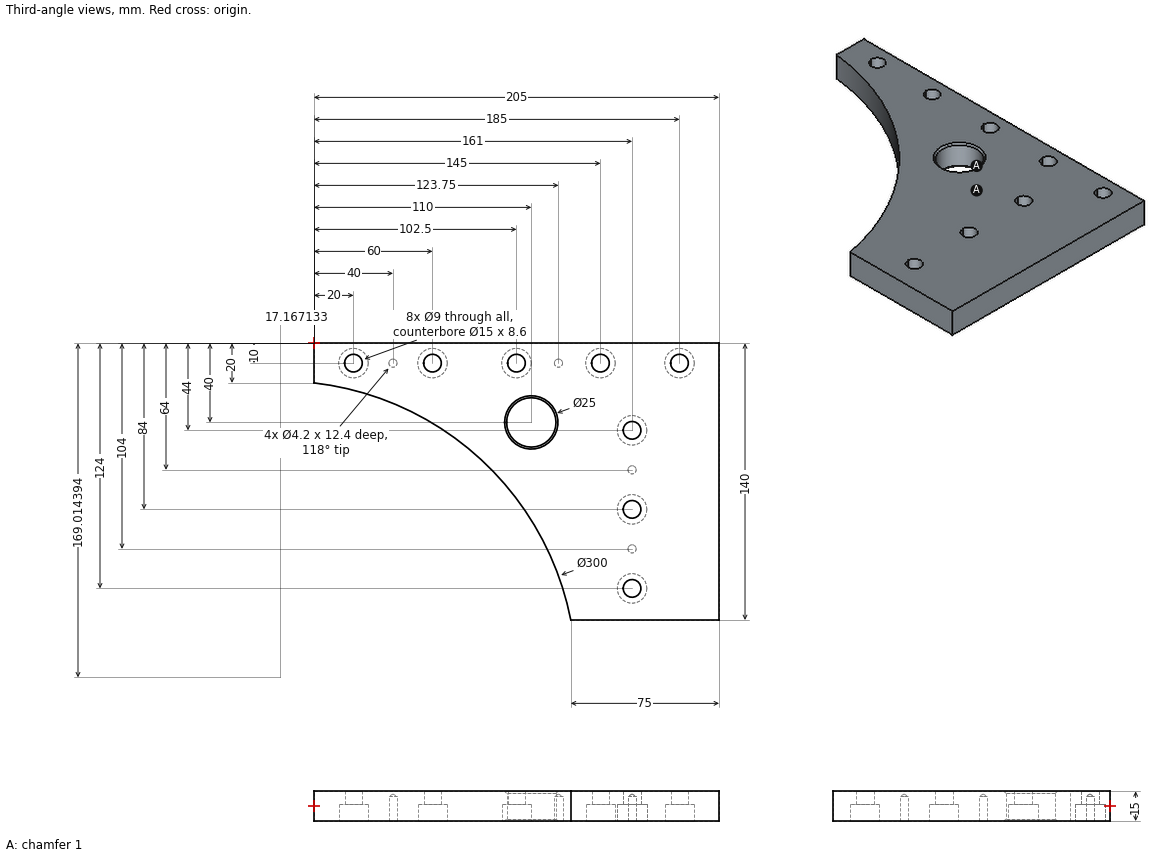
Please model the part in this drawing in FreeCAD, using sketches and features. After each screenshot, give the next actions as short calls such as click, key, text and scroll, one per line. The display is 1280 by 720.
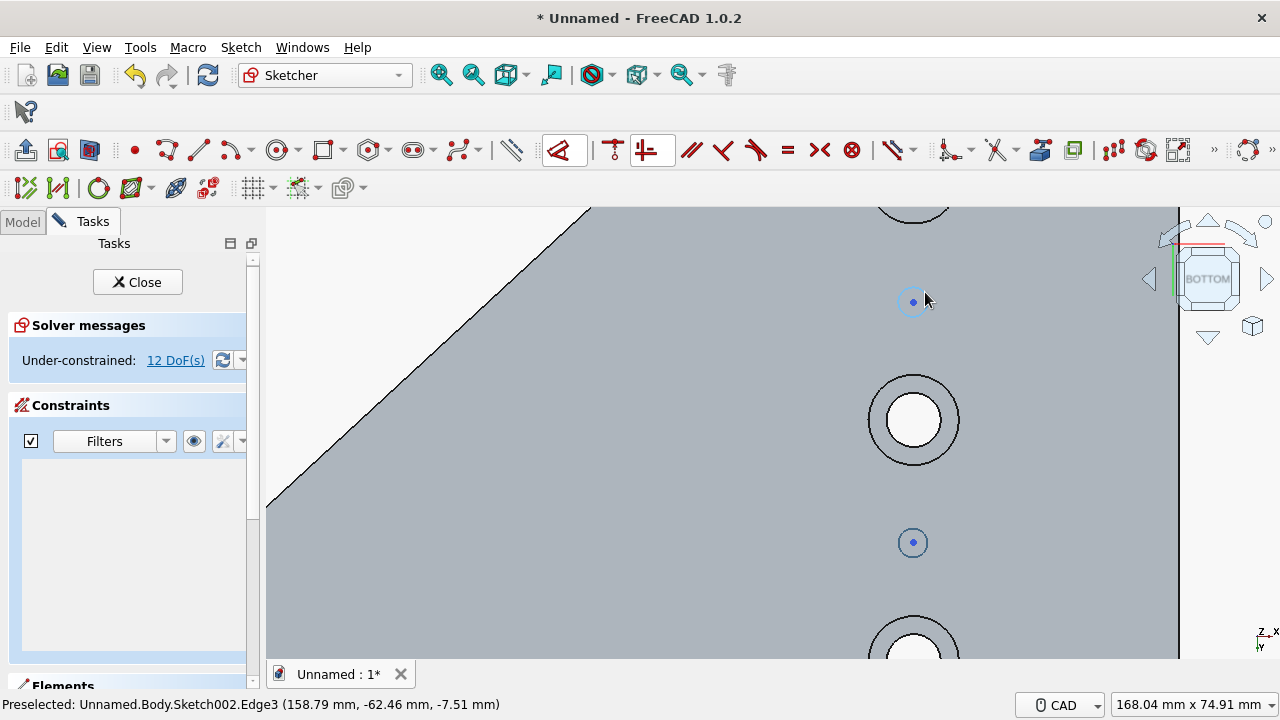
click(923, 292)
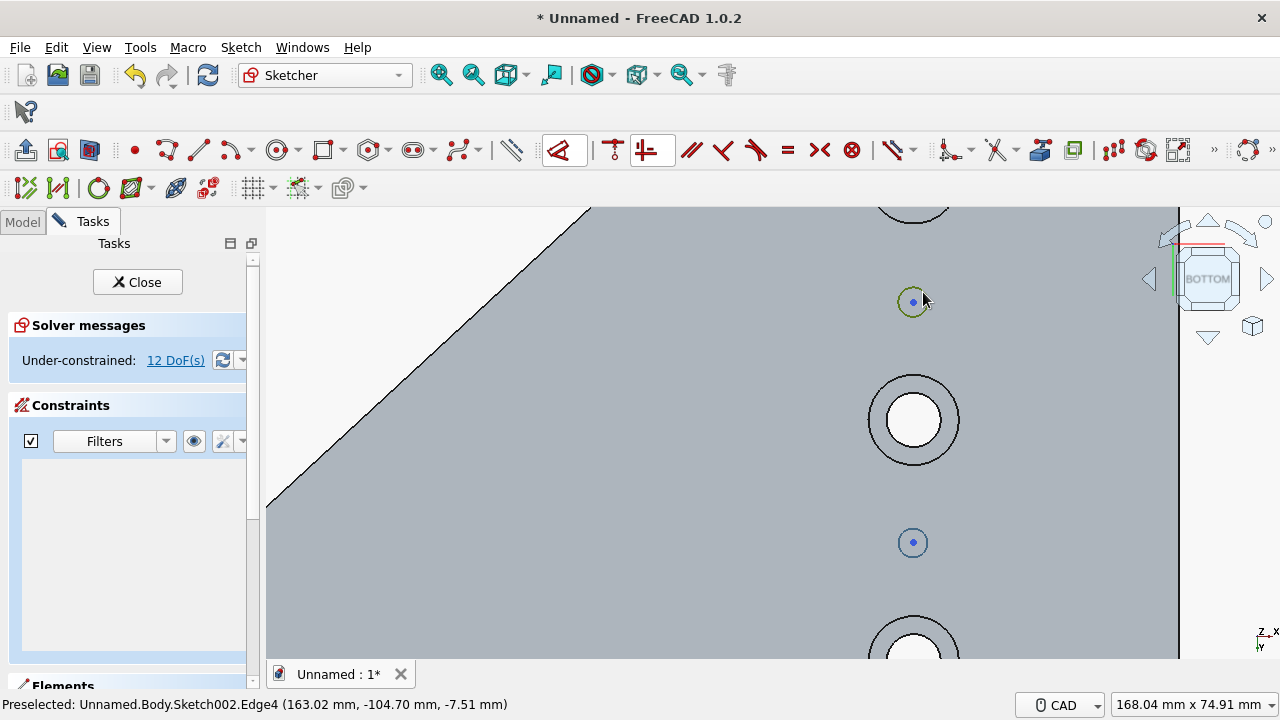
click(788, 150)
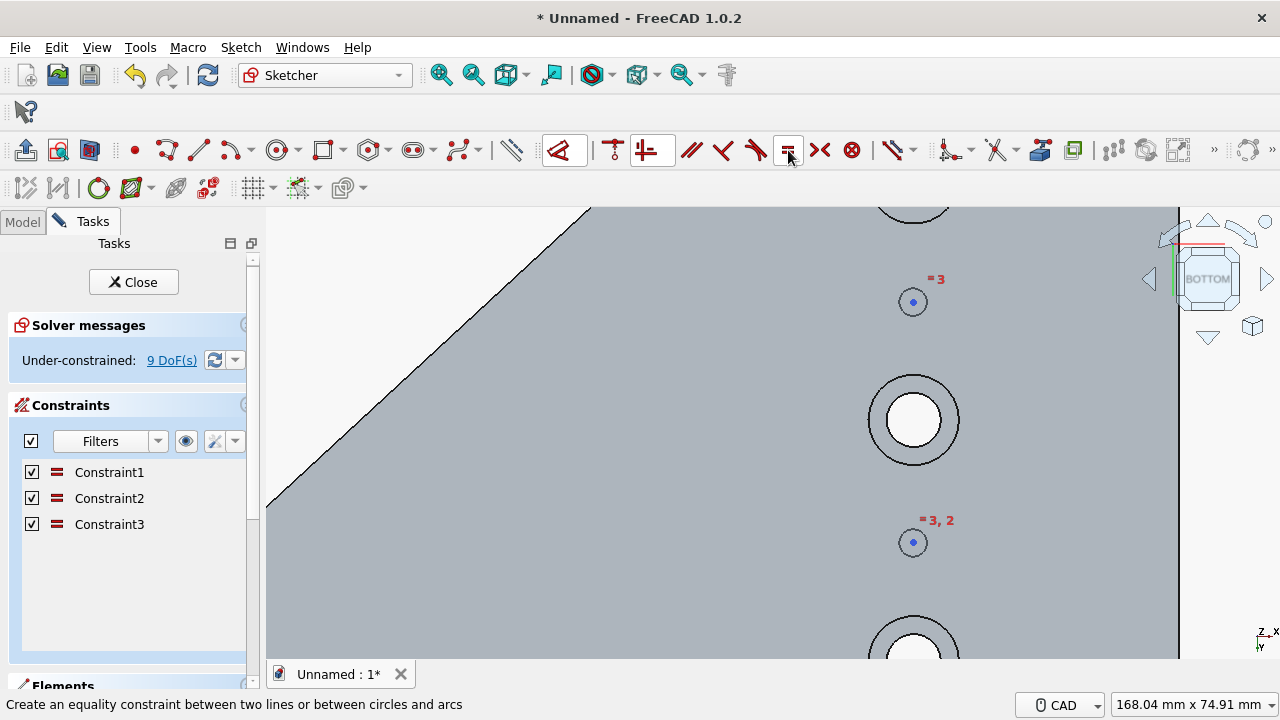
scroll(925, 291, down, 4)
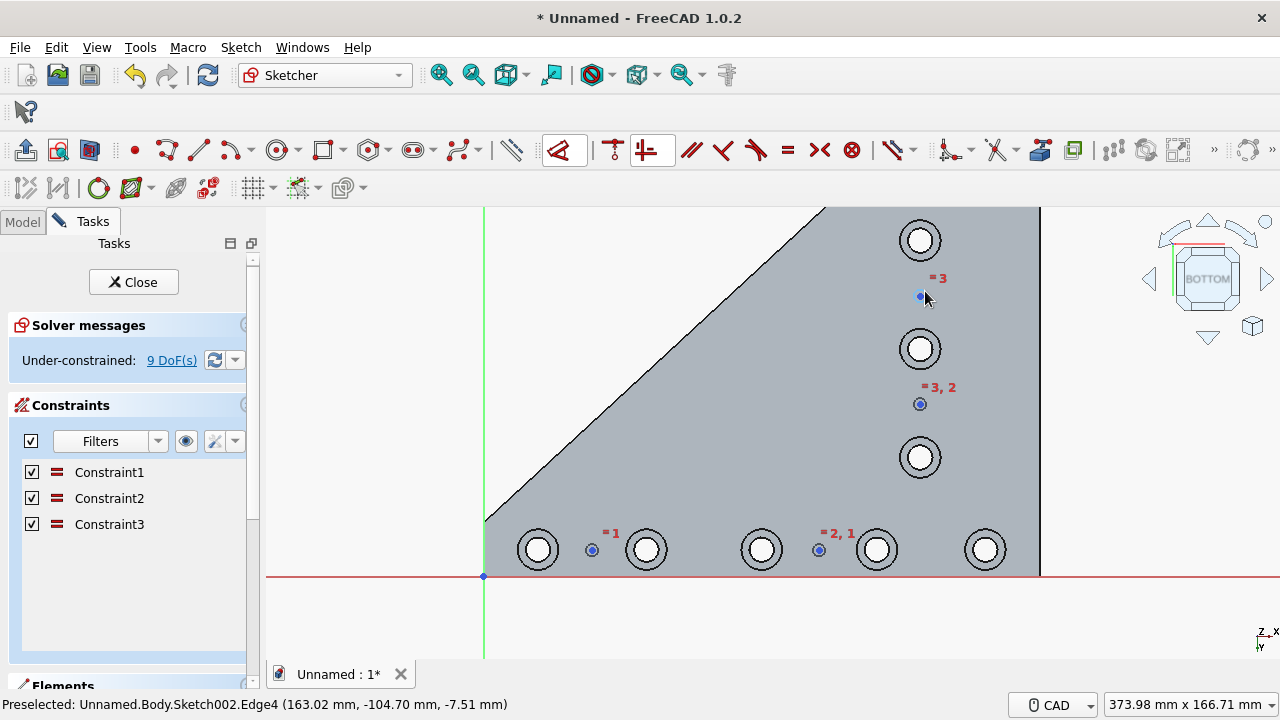
scroll(596, 546, up, 7)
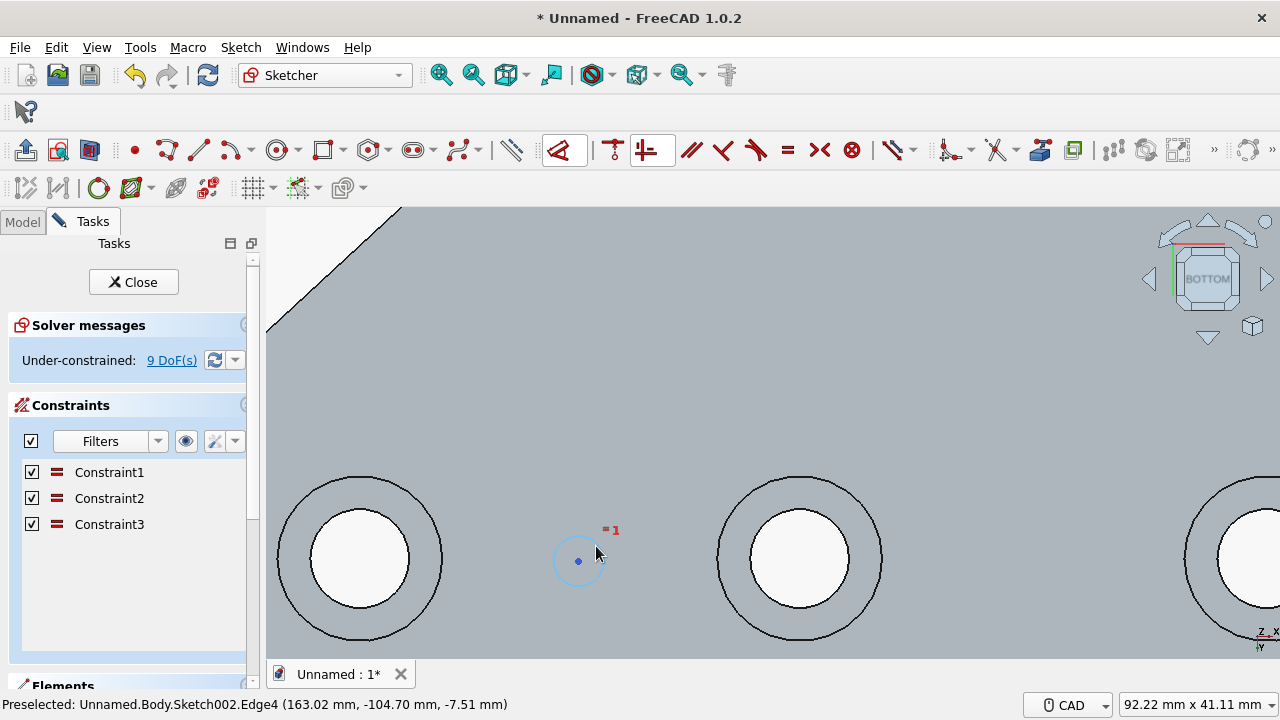
click(596, 544)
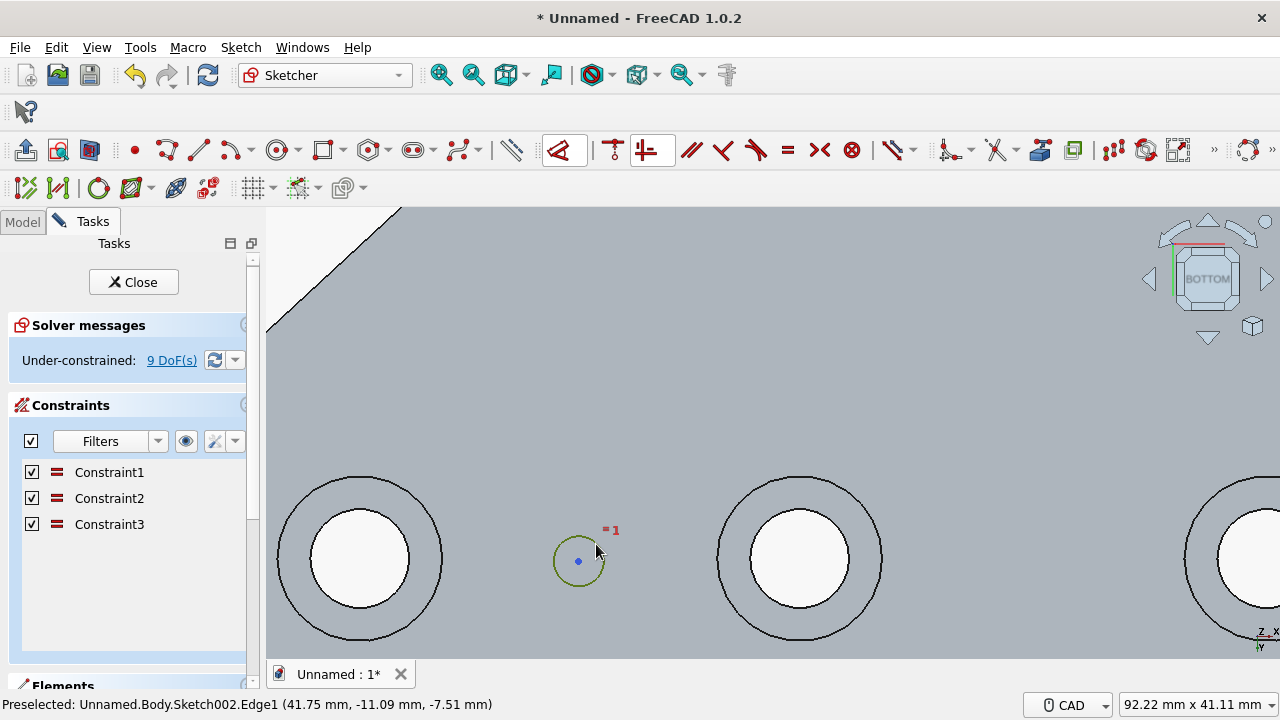
click(582, 150)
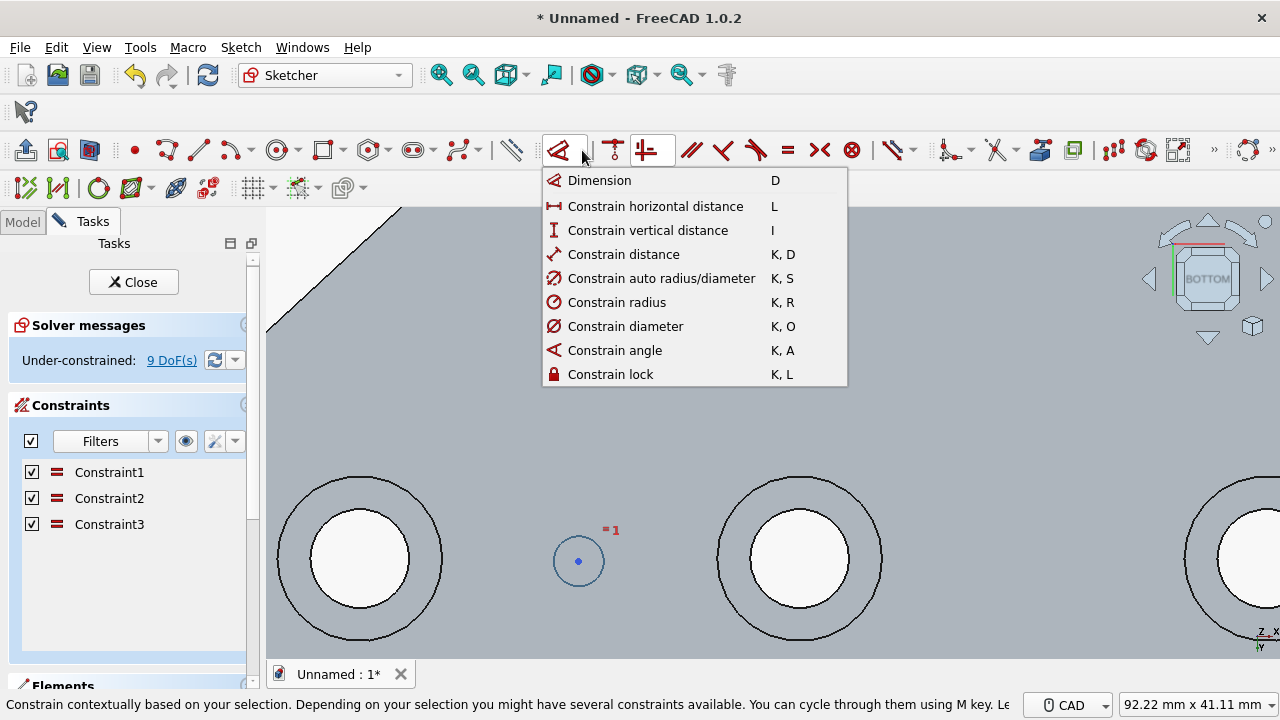
click(695, 326)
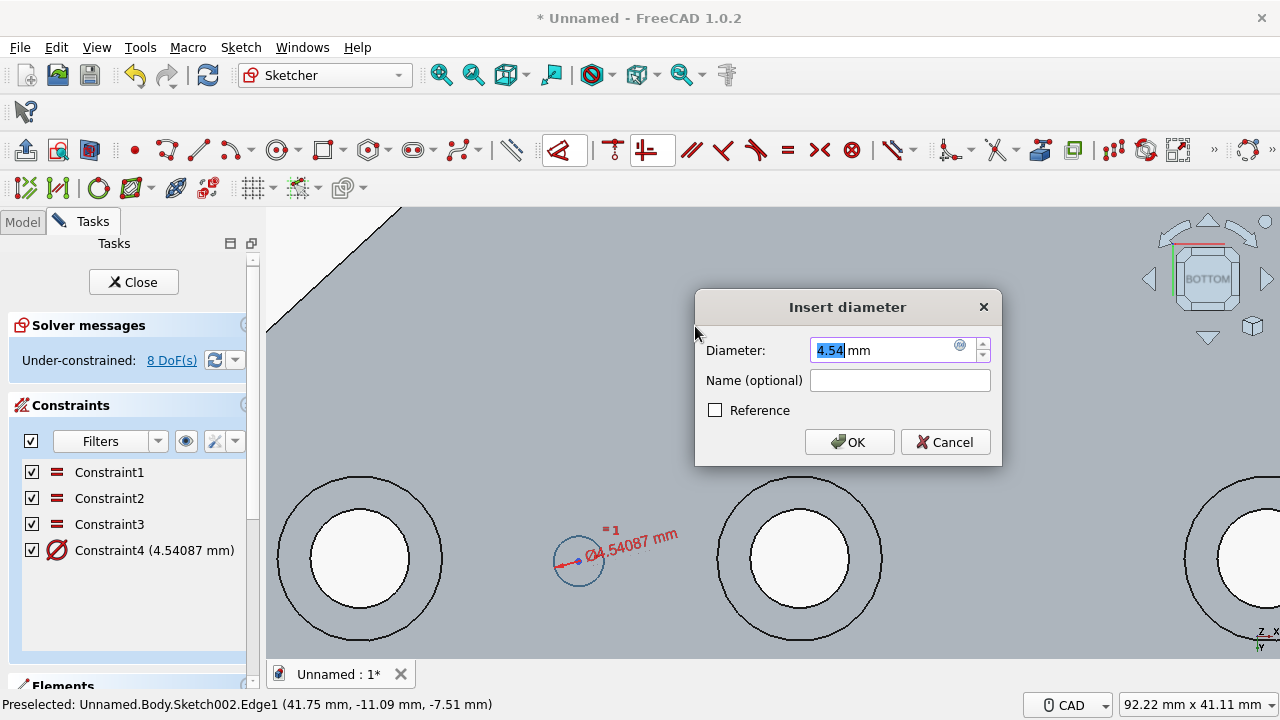
text(4.2)
key(Return)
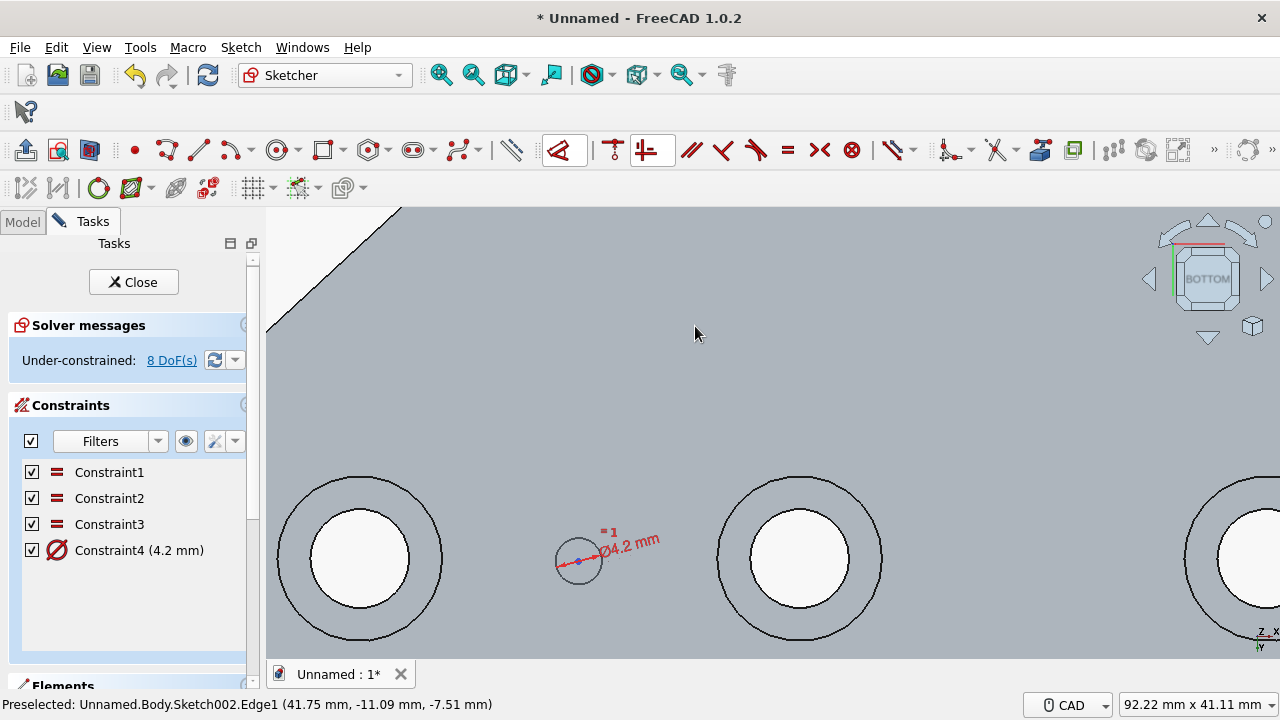
scroll(596, 547, down, 7)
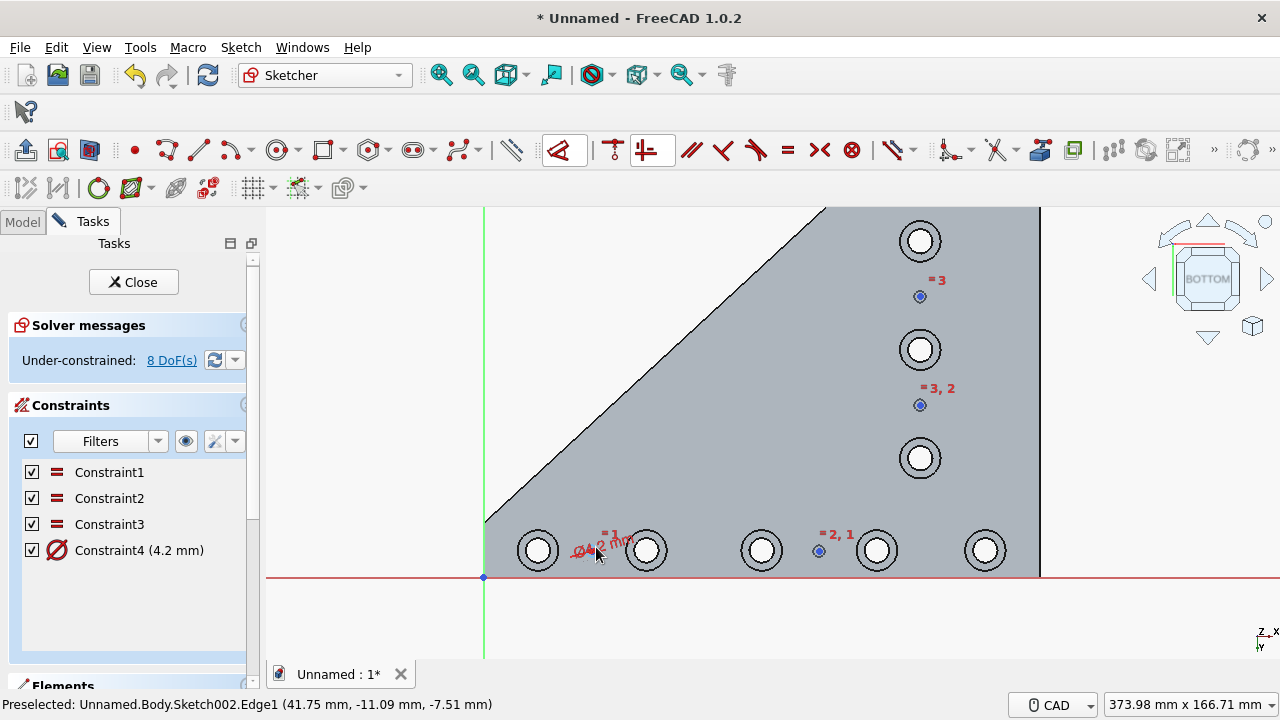
click(592, 551)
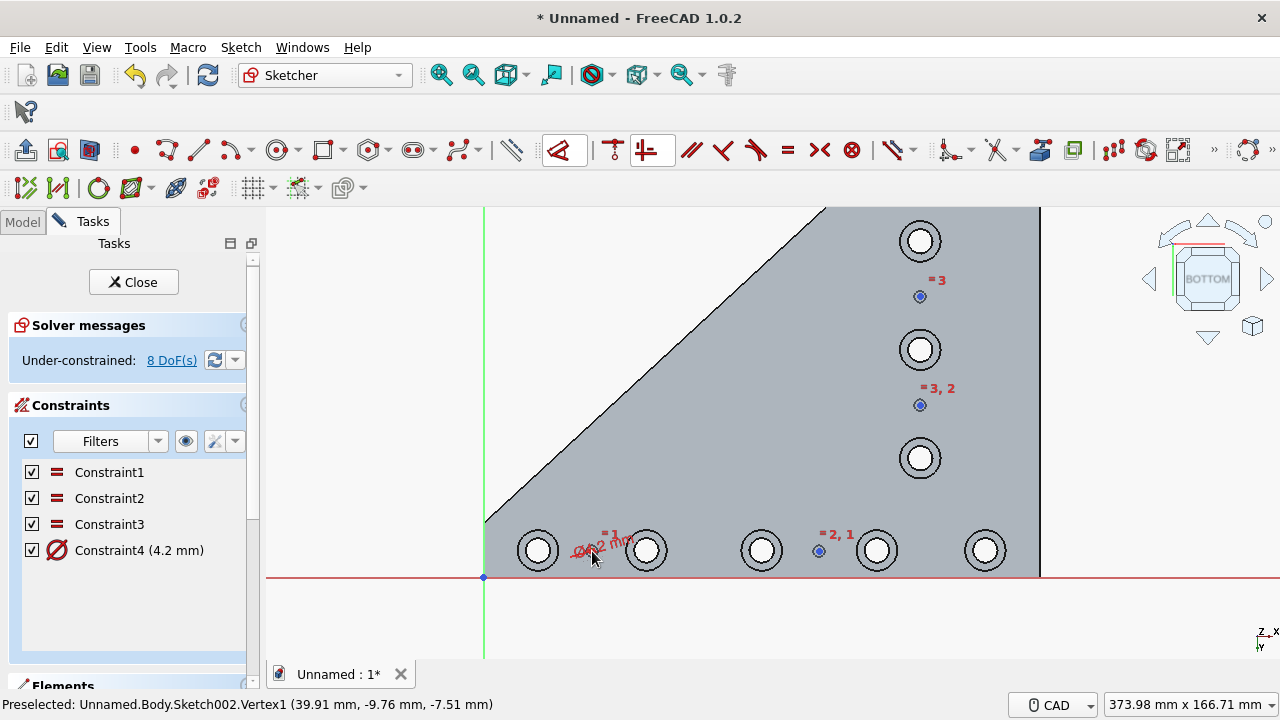
key(l)